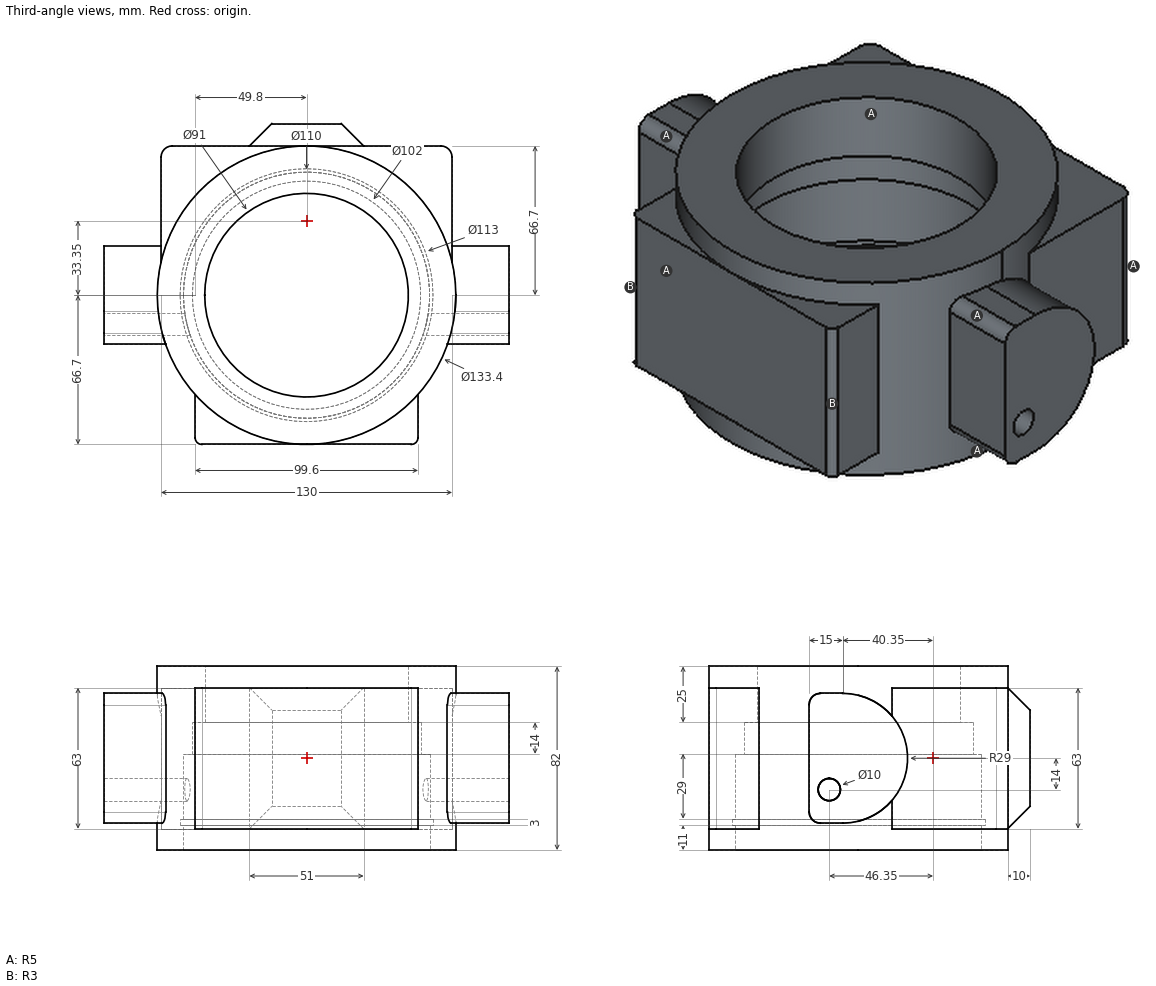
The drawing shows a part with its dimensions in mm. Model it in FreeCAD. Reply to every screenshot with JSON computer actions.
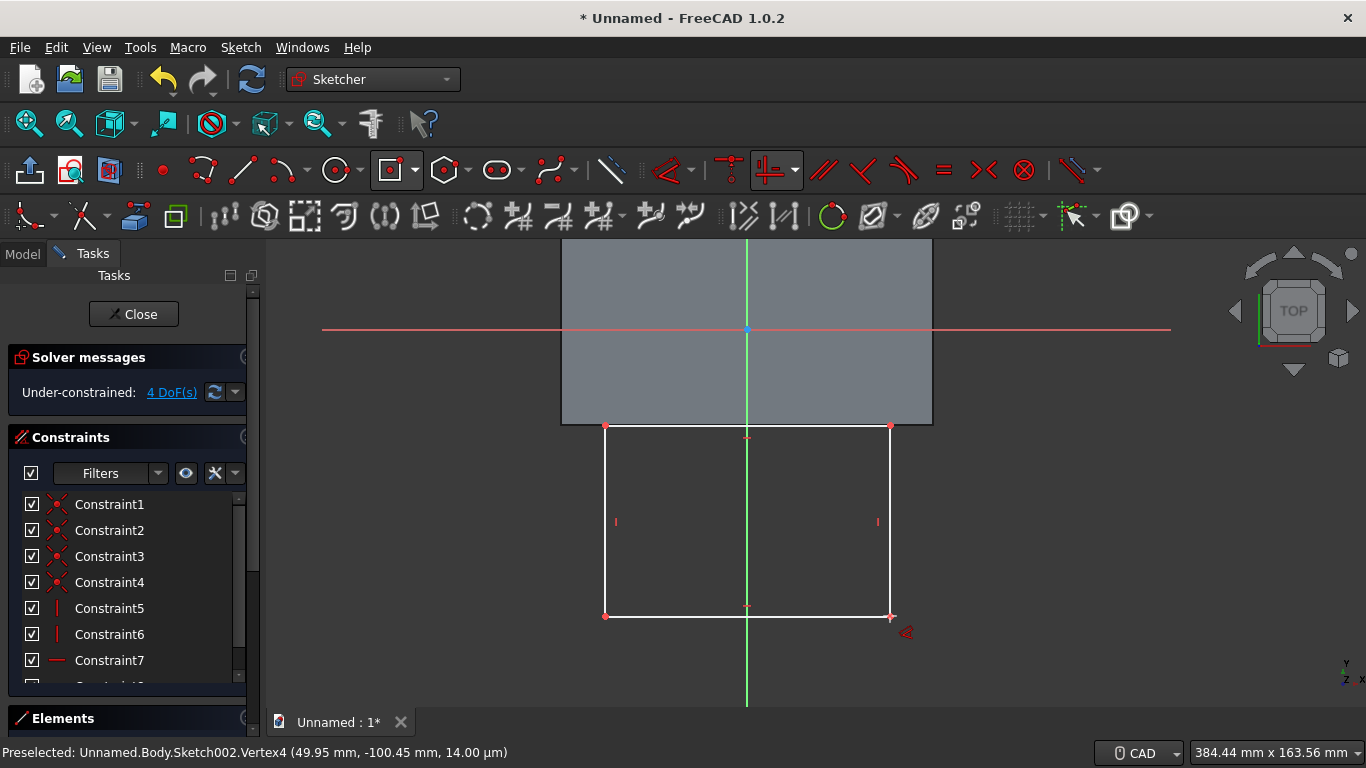
{"action": "left_click", "coordinate": [605, 483]}
{"action": "left_click", "coordinate": [571, 522]}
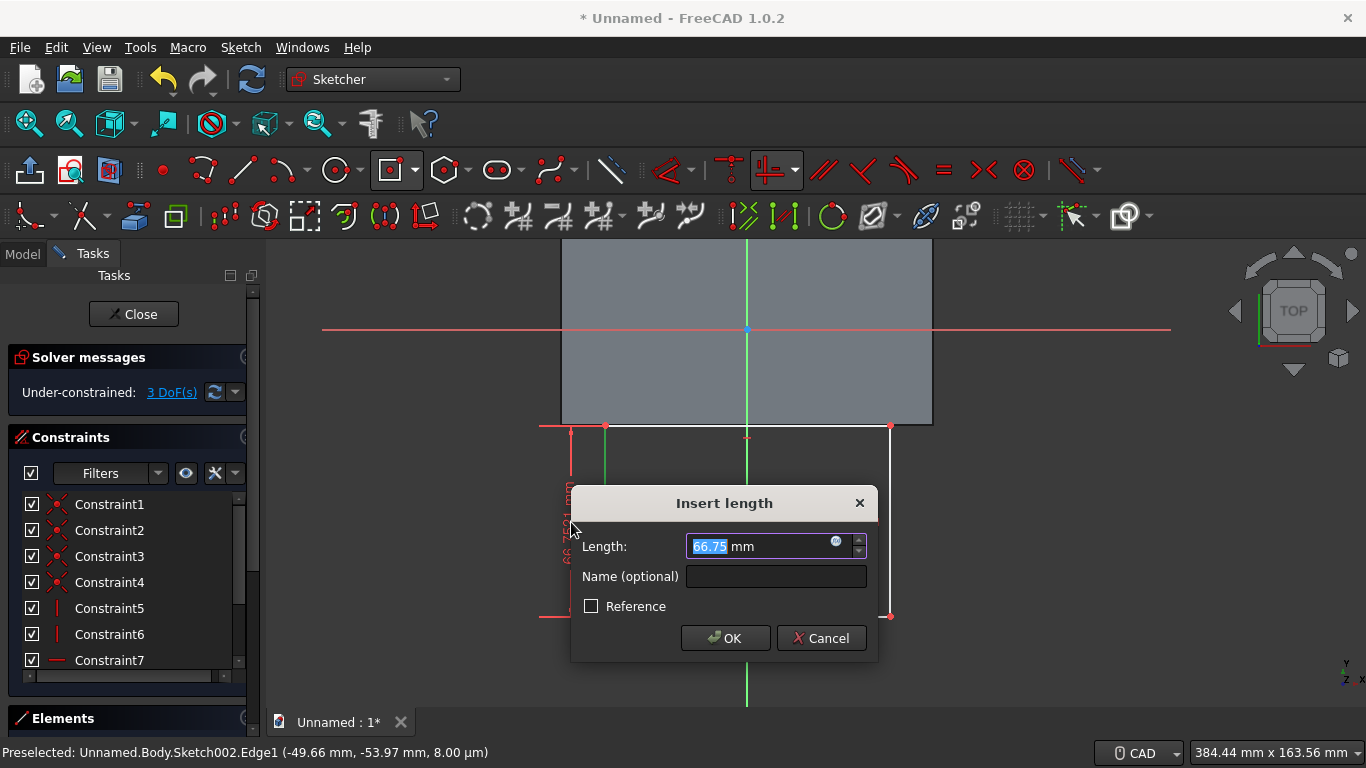
{"action": "type", "text": "66.7"}
{"action": "key", "text": "Return"}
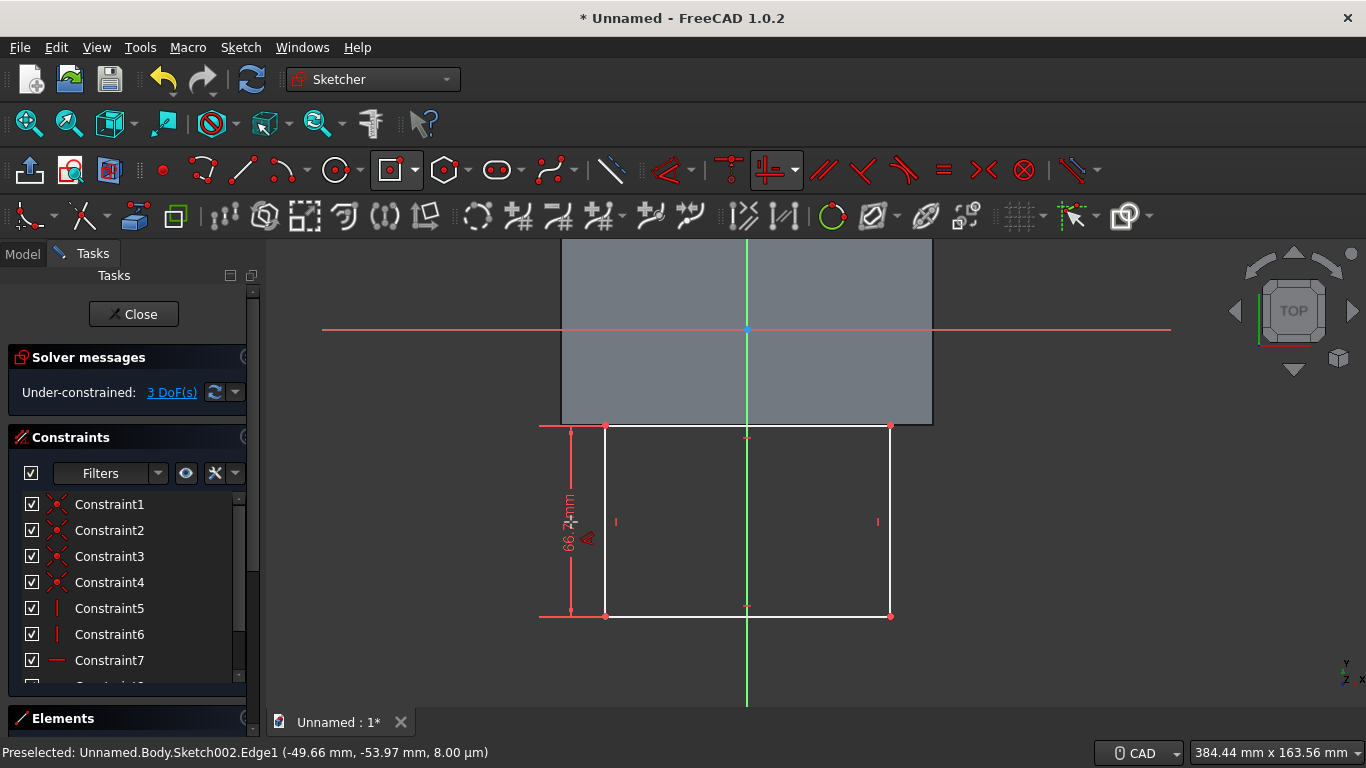
{"action": "left_click", "coordinate": [691, 617]}
{"action": "left_click", "coordinate": [682, 651]}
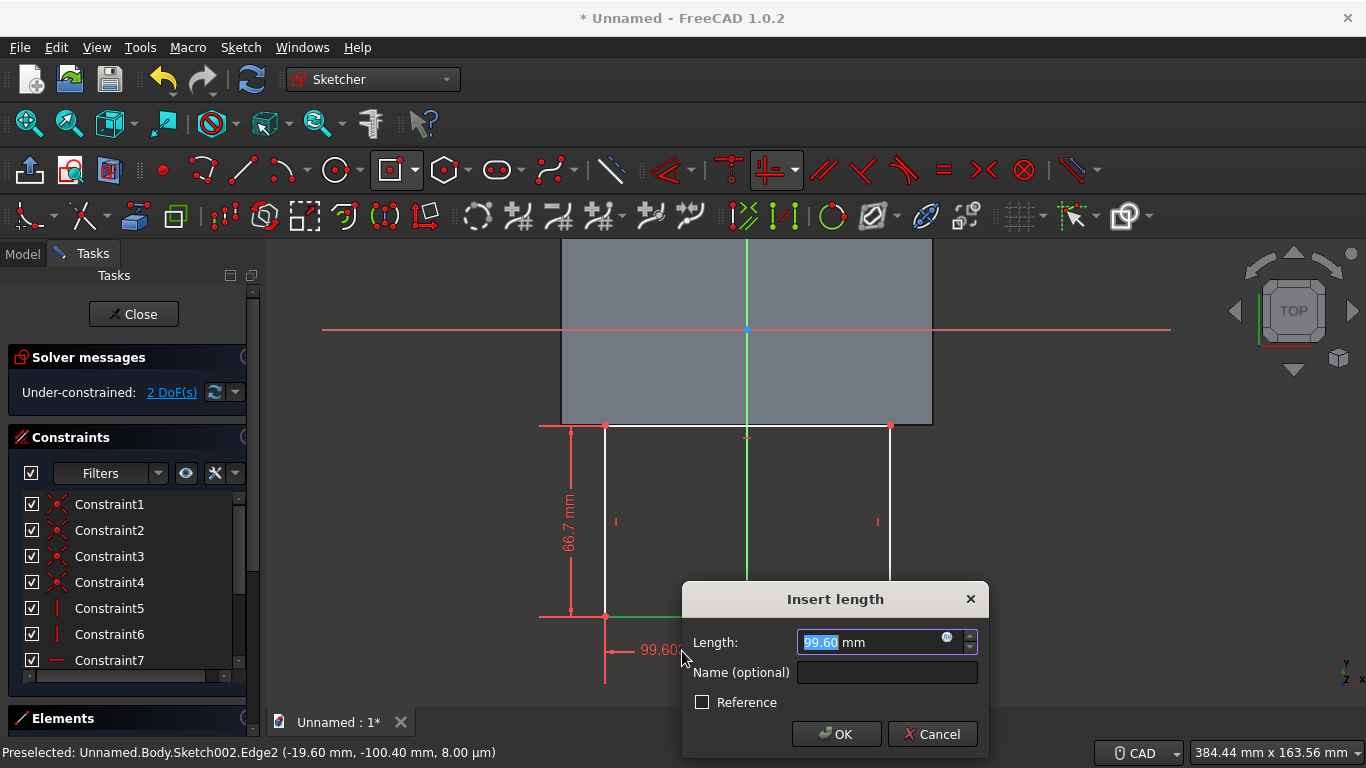
{"action": "type", "text": "99.6"}
{"action": "key", "text": "Return"}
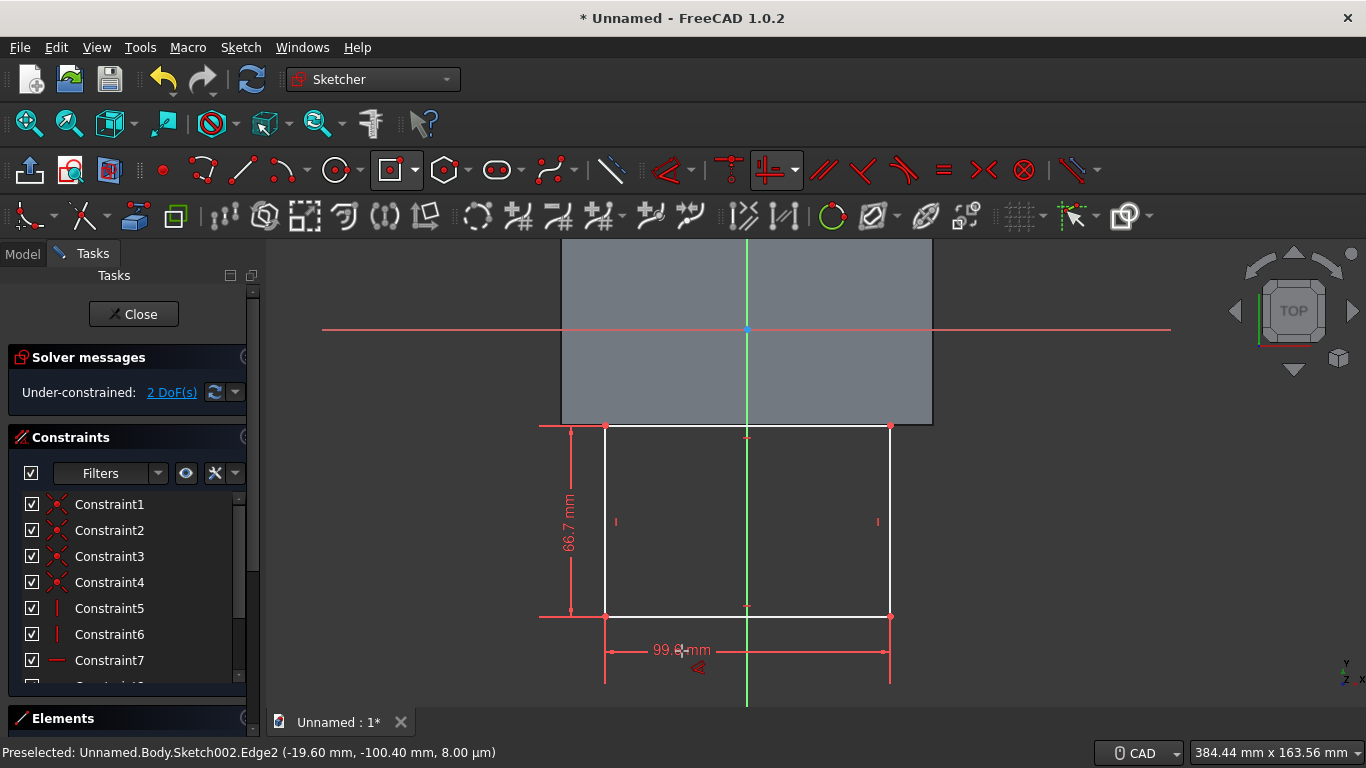
{"action": "left_click", "coordinate": [605, 426]}
{"action": "left_click", "coordinate": [676, 296]}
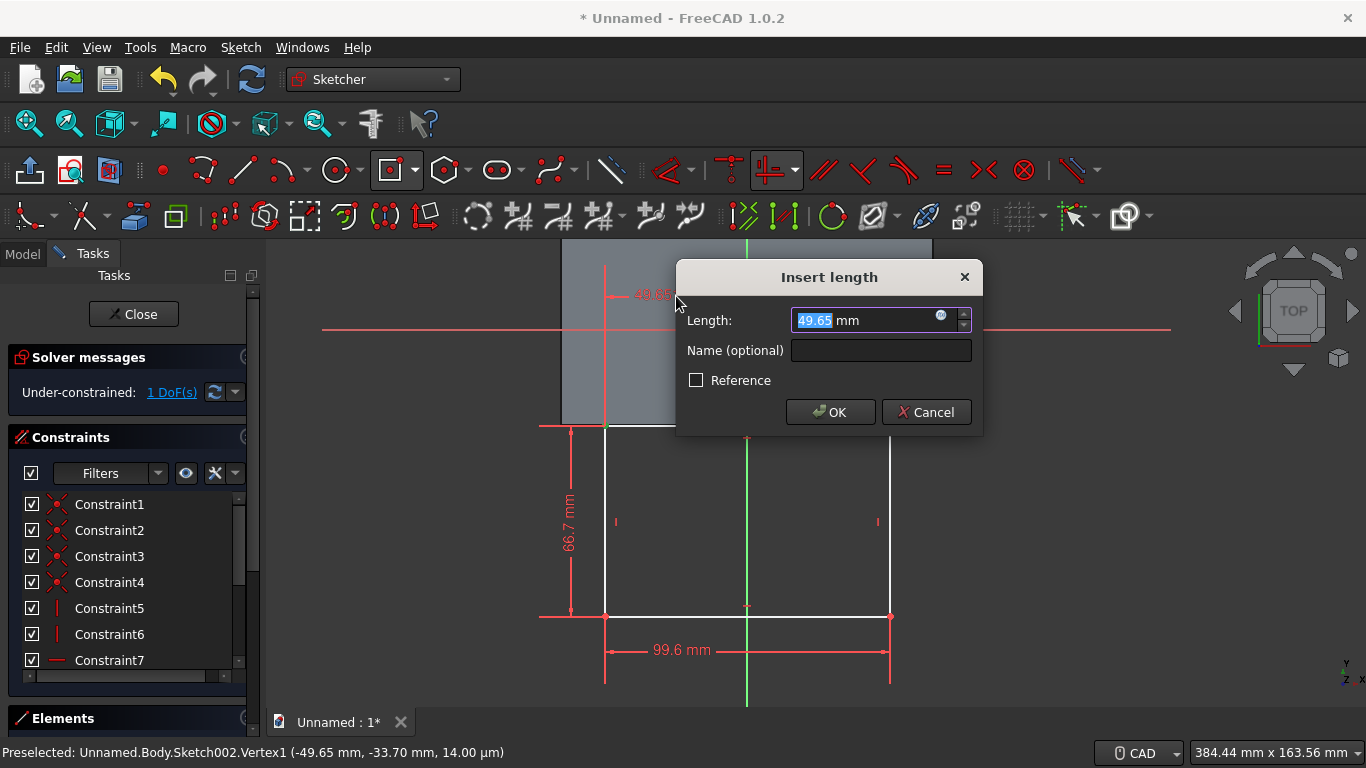
{"action": "type", "text": "49.8"}
{"action": "key", "text": "Return"}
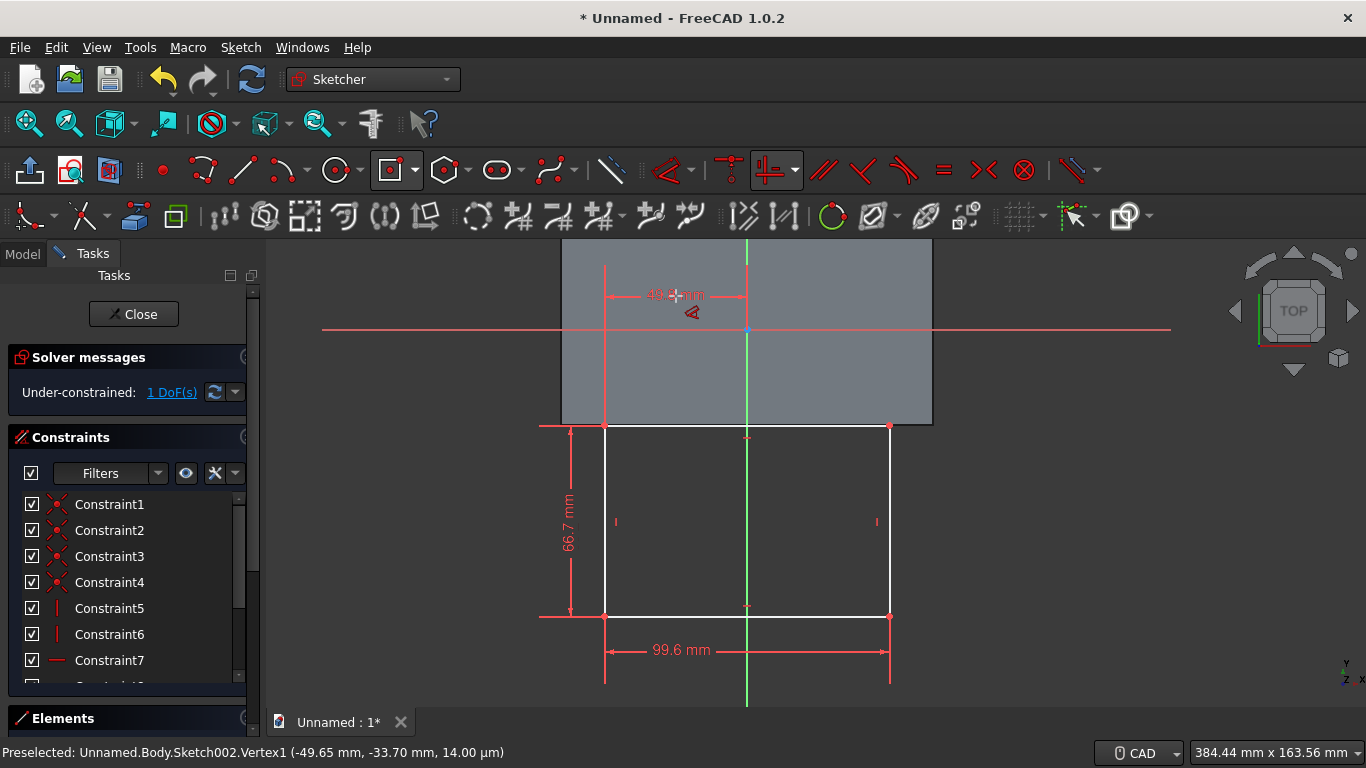
{"action": "left_click", "coordinate": [605, 426]}
{"action": "left_click", "coordinate": [571, 378]}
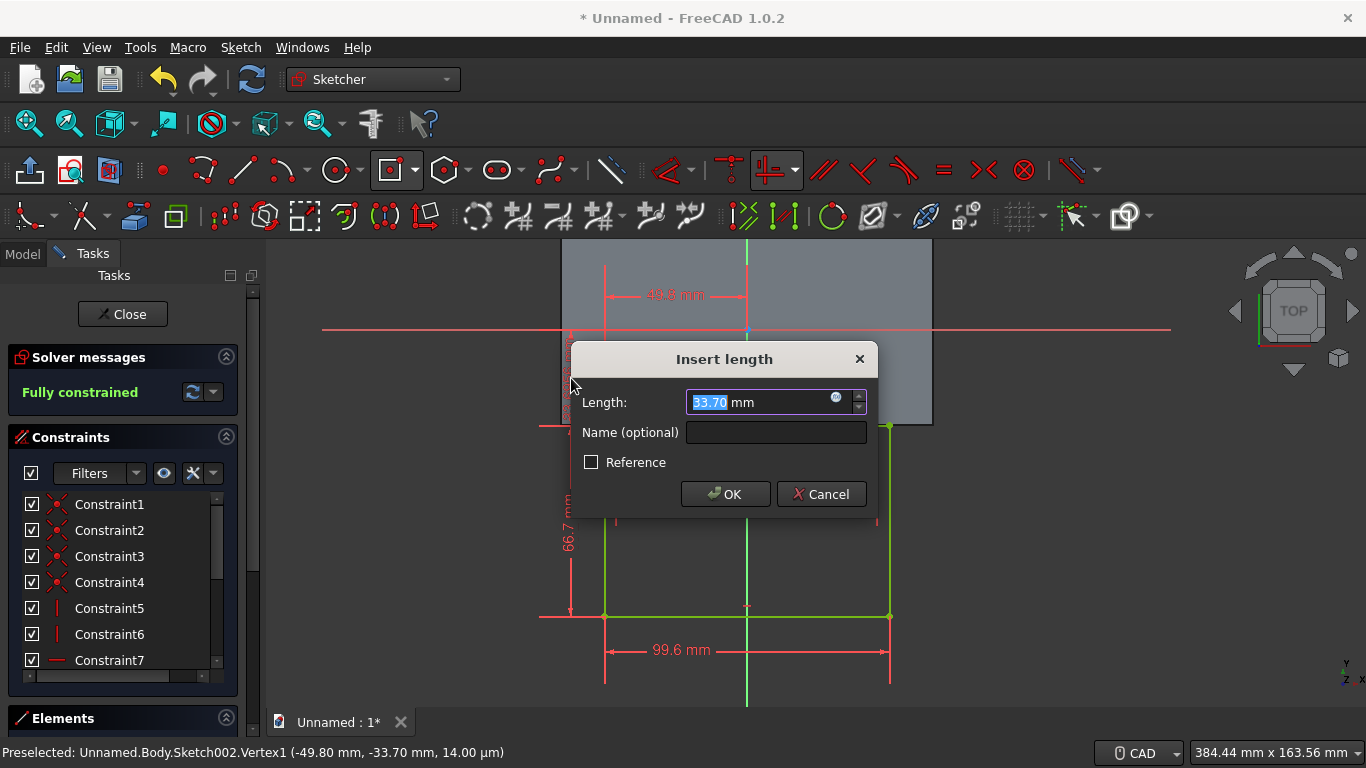
{"action": "type", "text": "33.35"}
{"action": "key", "text": "Return"}
{"action": "key", "text": "Escape"}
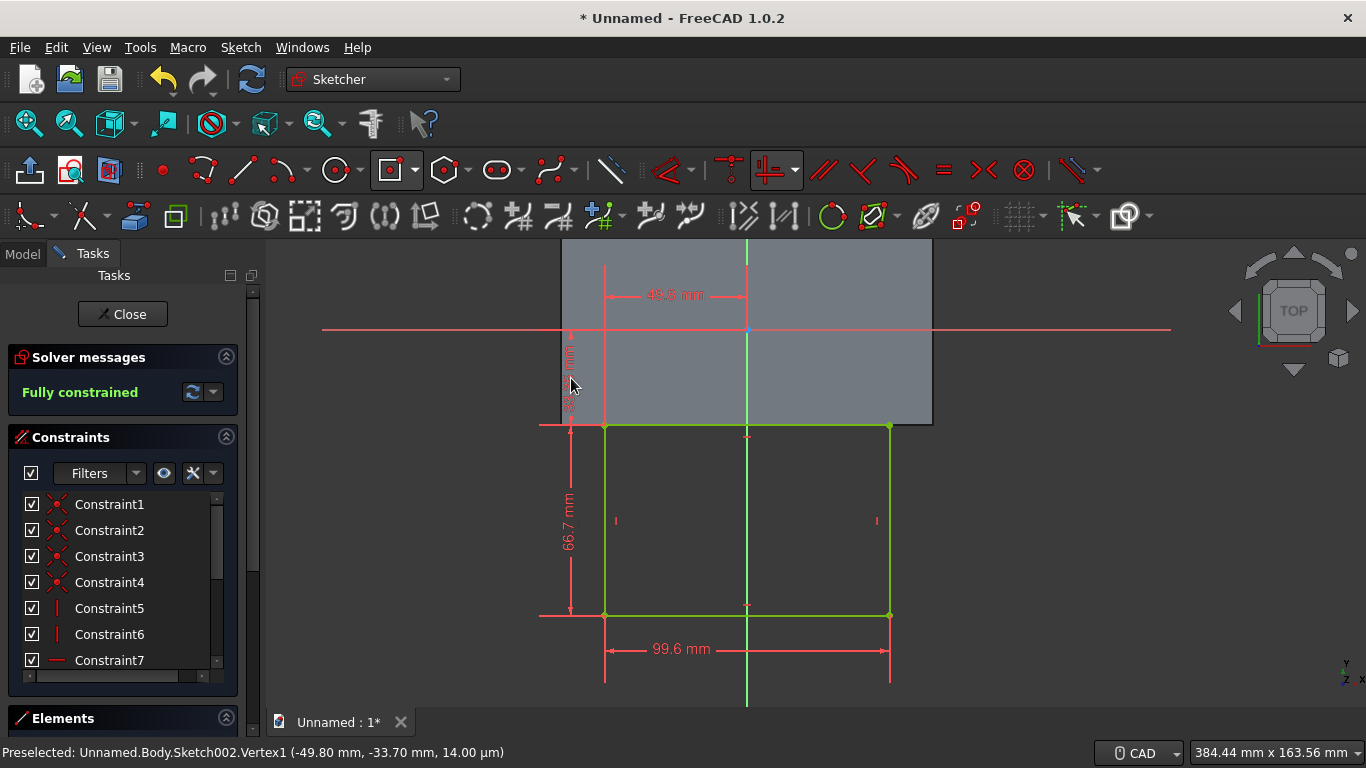
{"action": "left_click", "coordinate": [123, 314]}